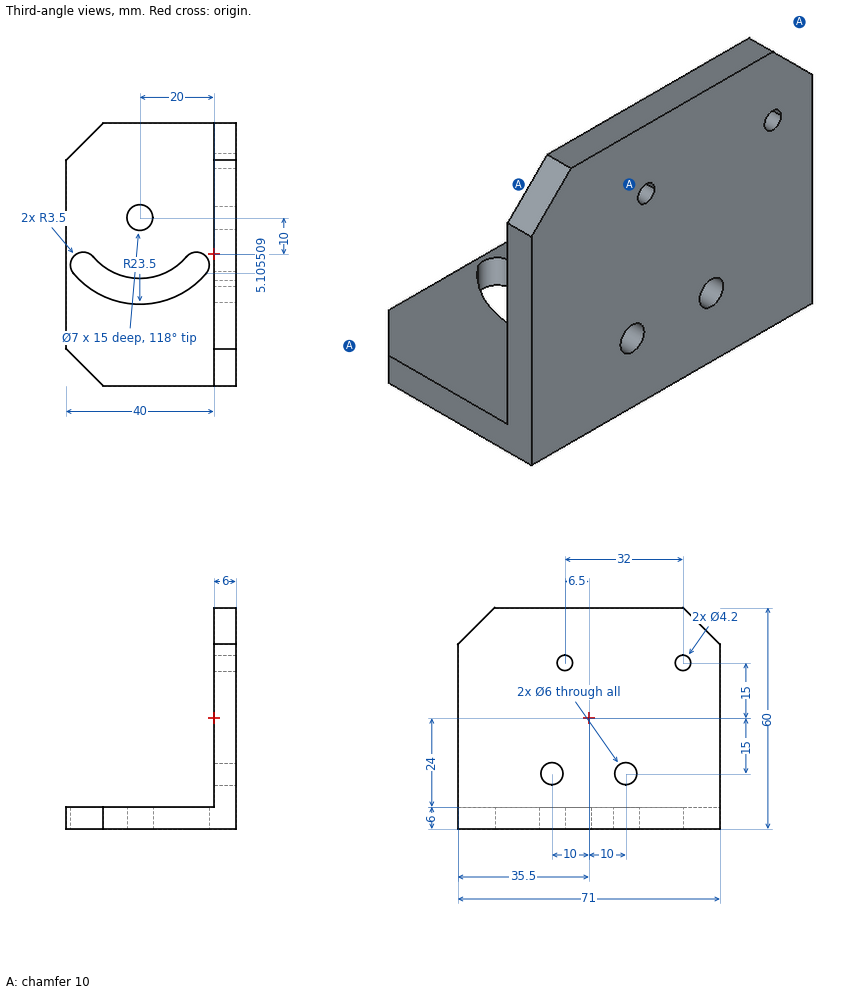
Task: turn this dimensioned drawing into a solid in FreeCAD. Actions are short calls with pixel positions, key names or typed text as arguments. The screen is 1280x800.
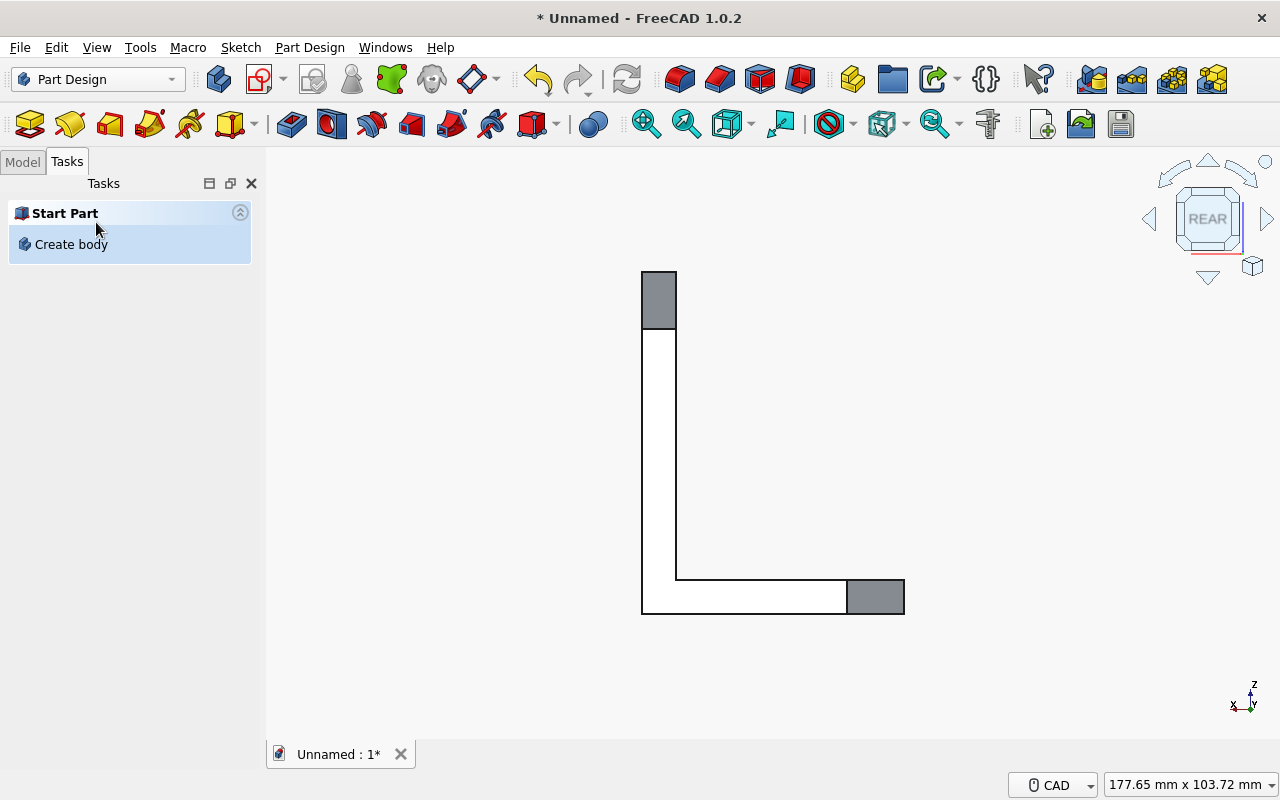
key(0)